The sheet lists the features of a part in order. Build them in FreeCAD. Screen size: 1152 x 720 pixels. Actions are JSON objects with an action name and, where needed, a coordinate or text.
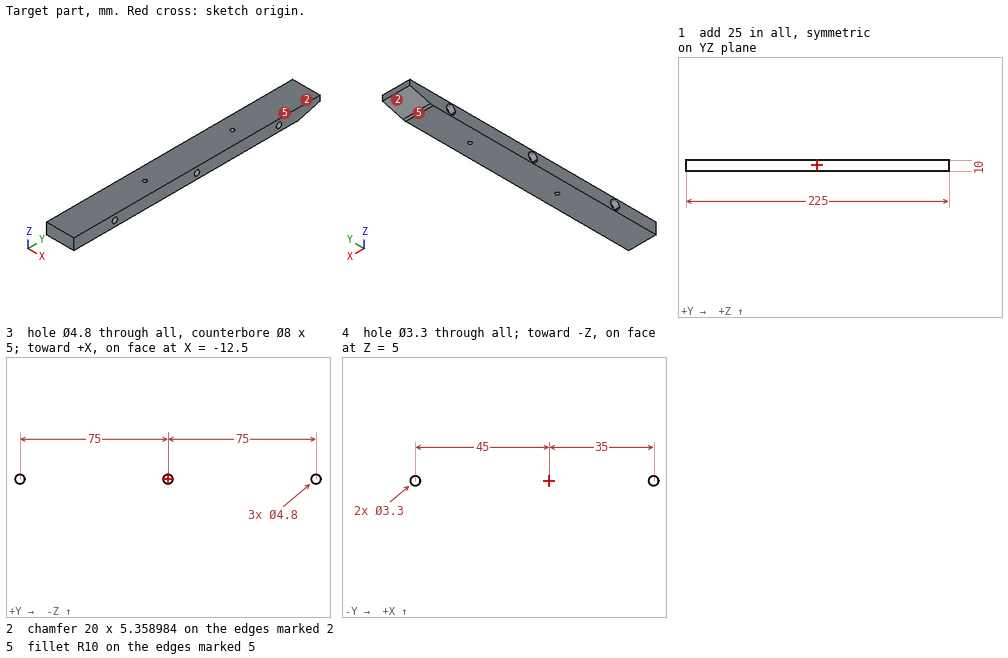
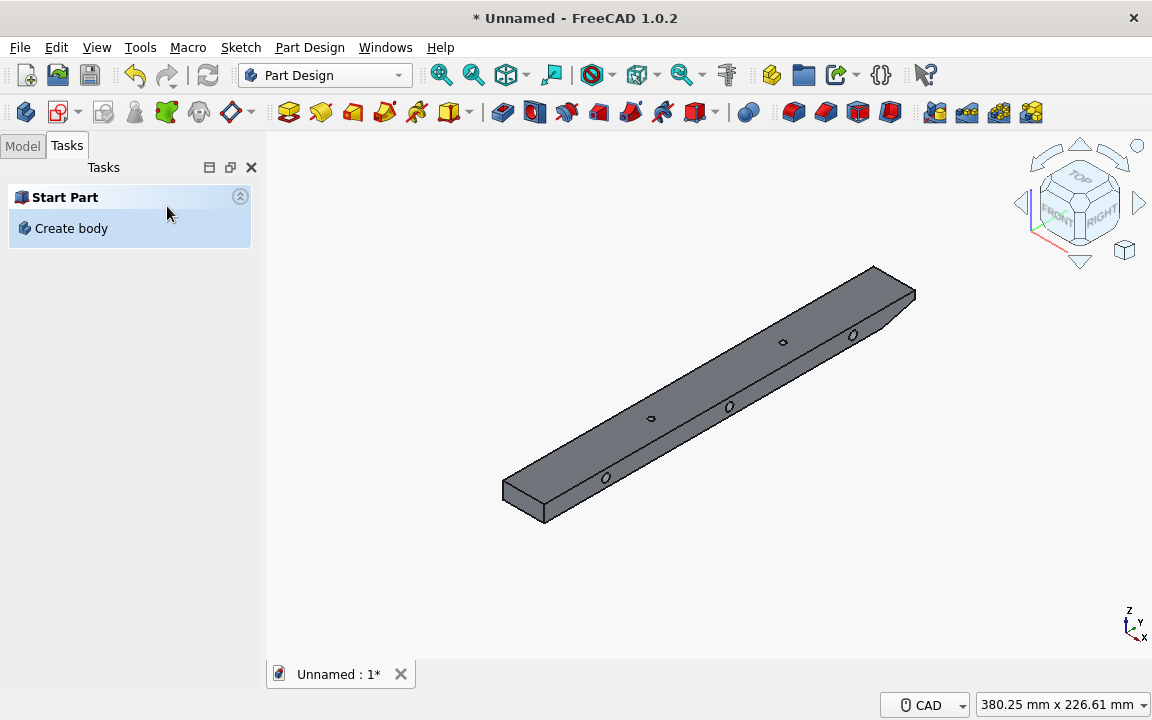
{"action": "key", "text": "2"}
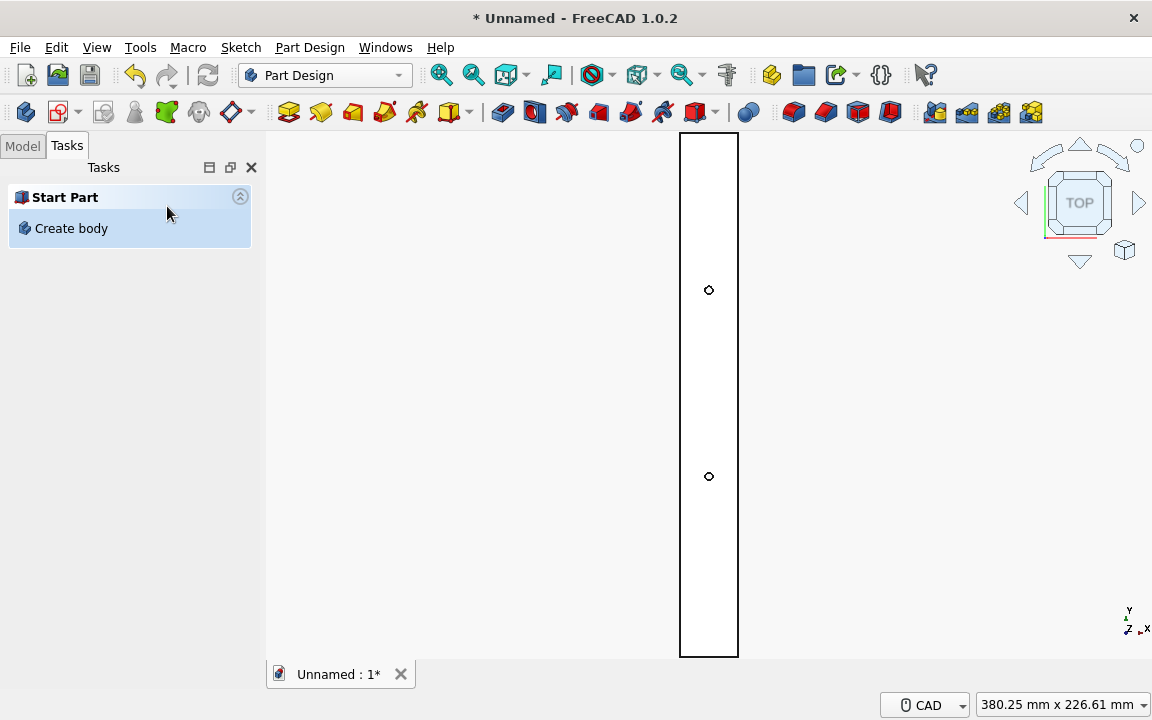
{"action": "key", "text": "0"}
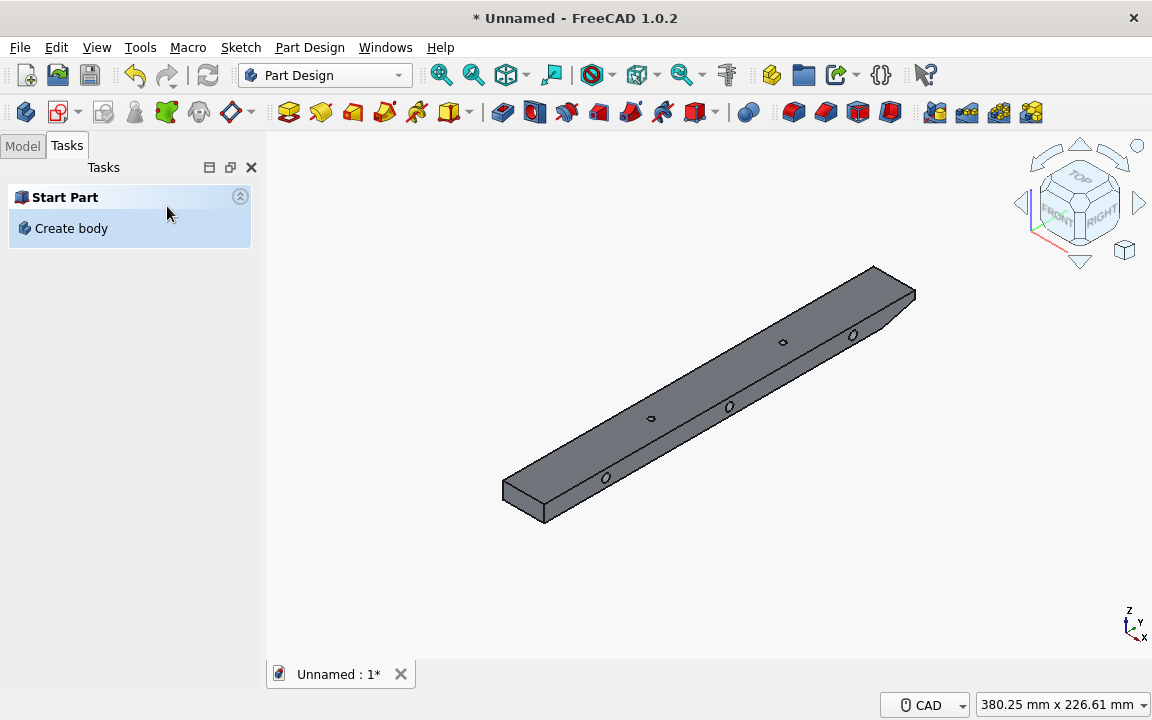
{"action": "key", "text": "1"}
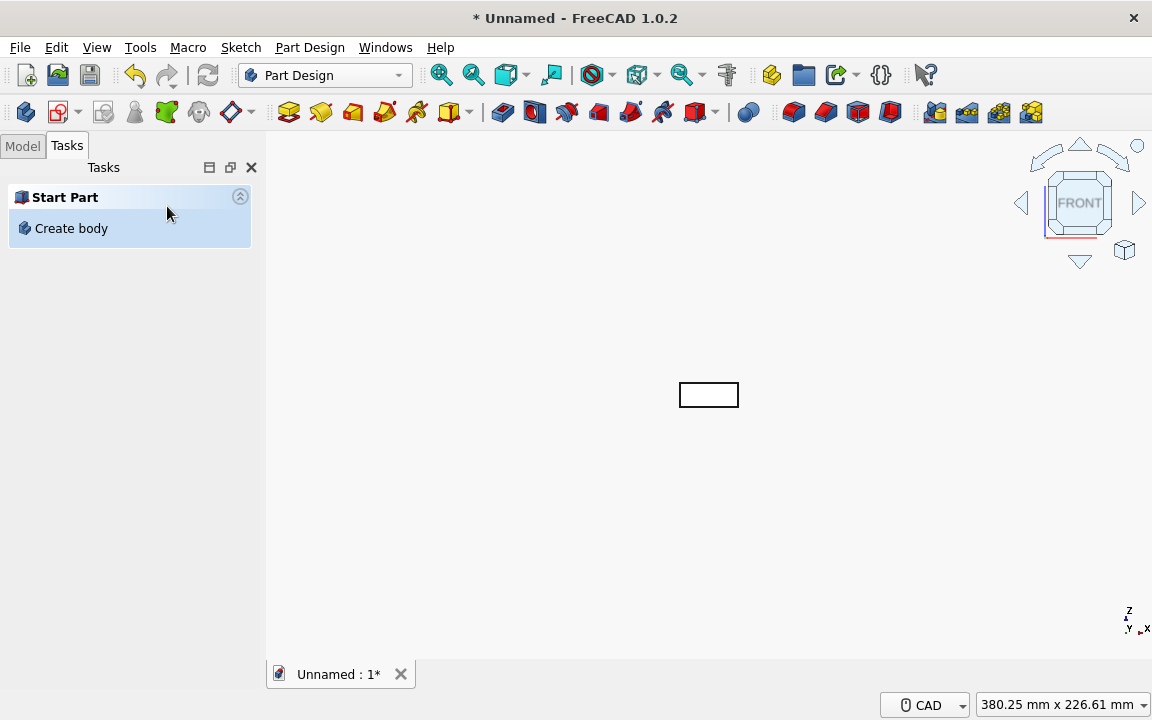
{"action": "left_click", "coordinate": [442, 76]}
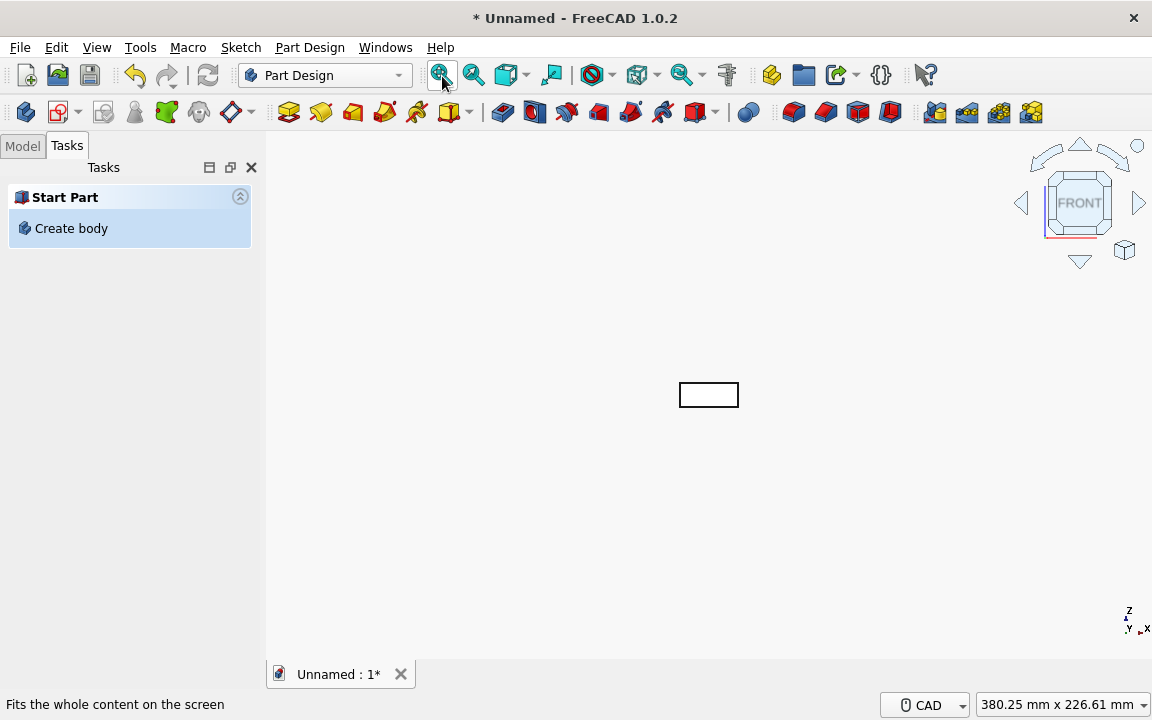
{"action": "key", "text": "3"}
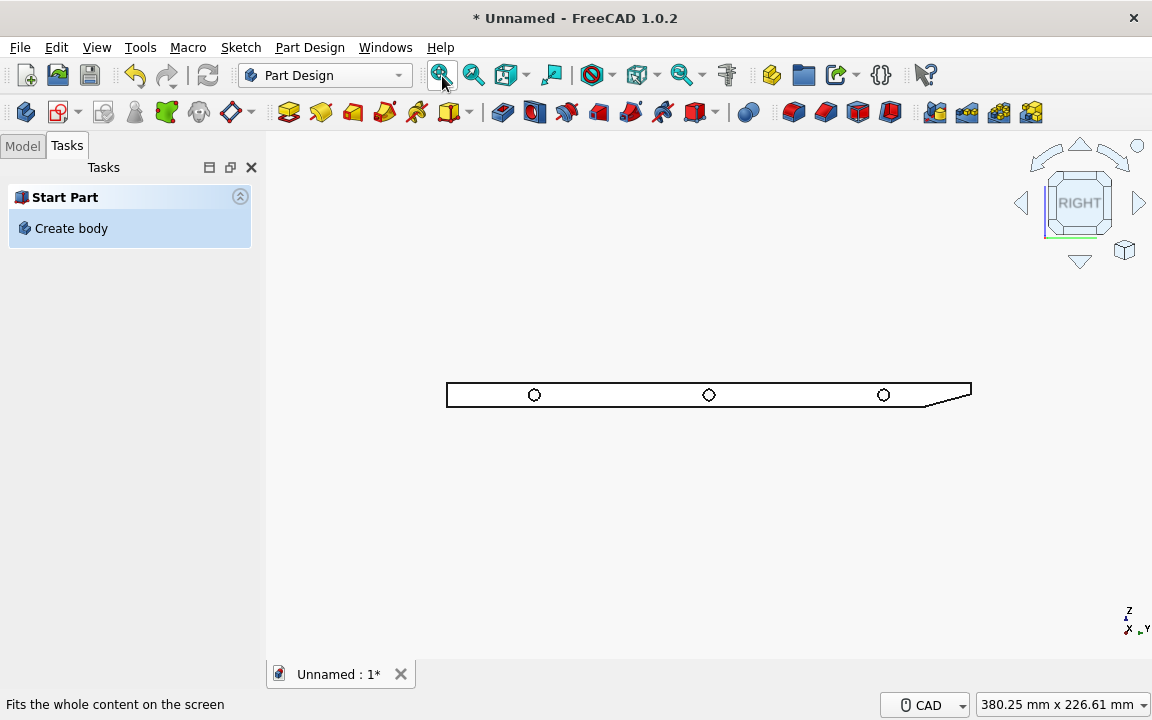
{"action": "key", "text": "5"}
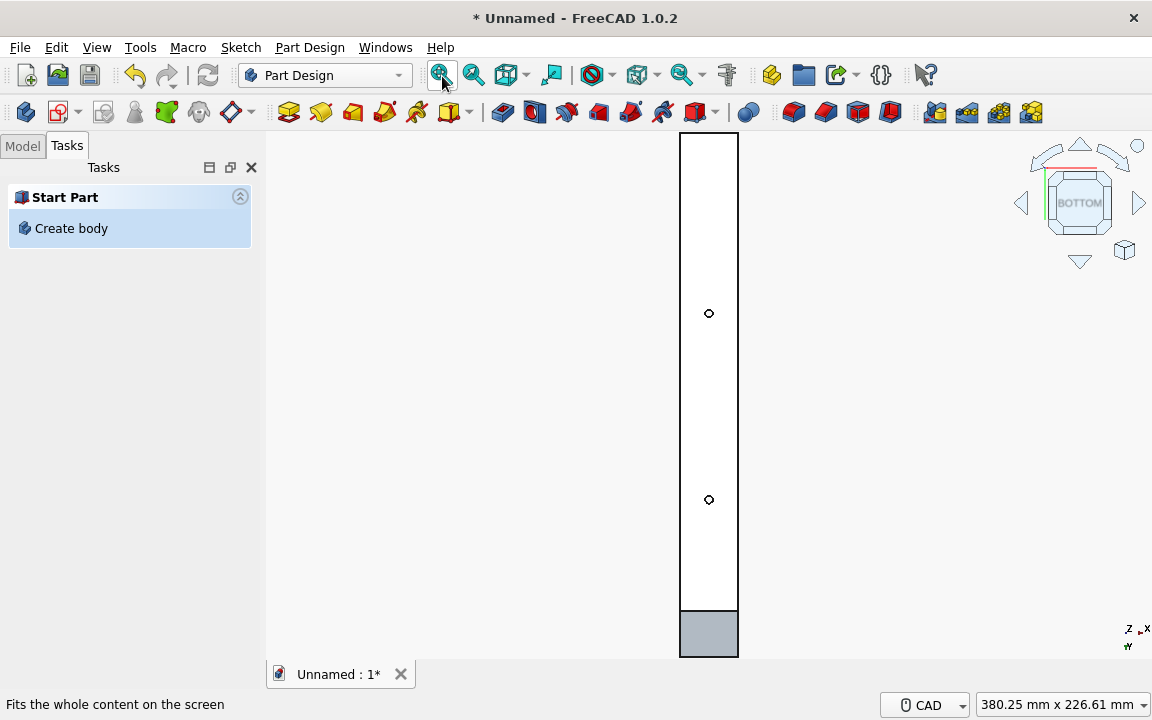
{"action": "left_click", "coordinate": [709, 610]}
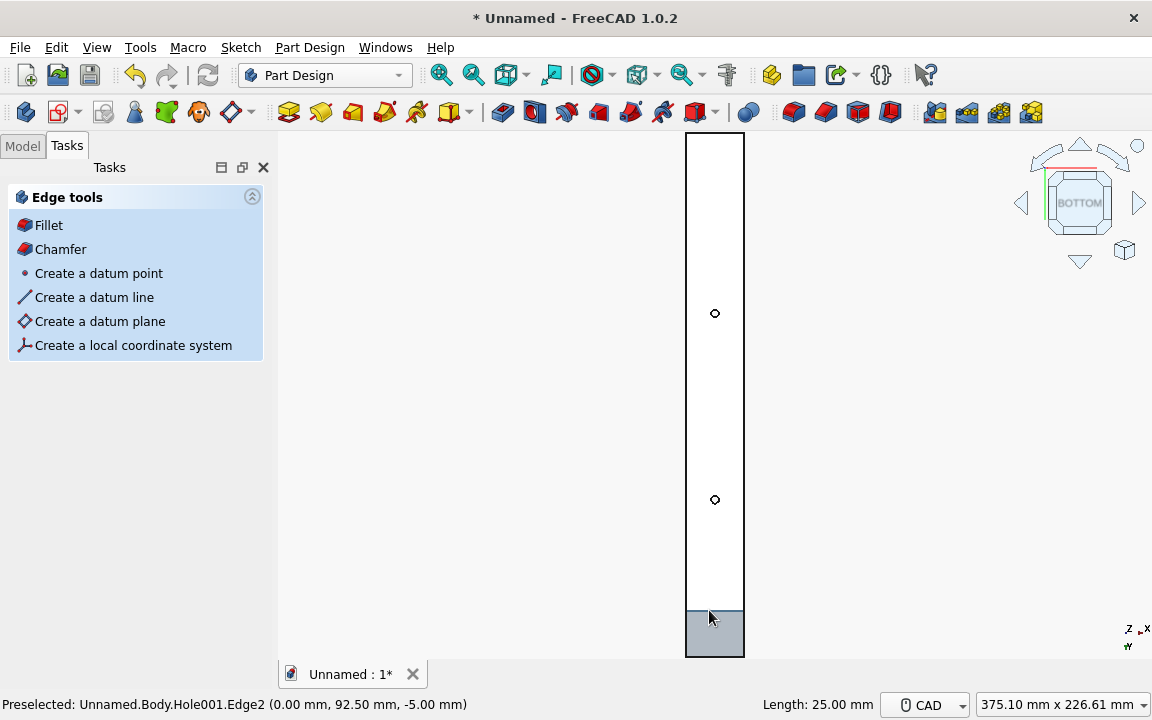
{"action": "left_click", "coordinate": [794, 112]}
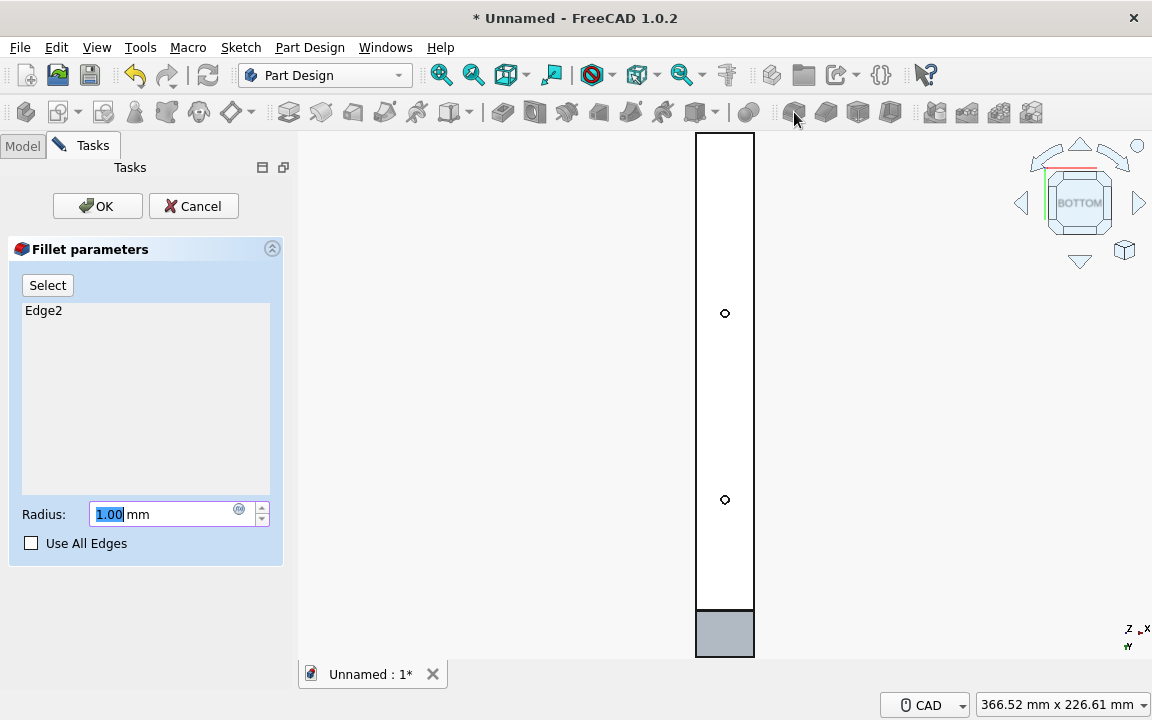
{"action": "type", "text": "10"}
{"action": "key", "text": "Tab"}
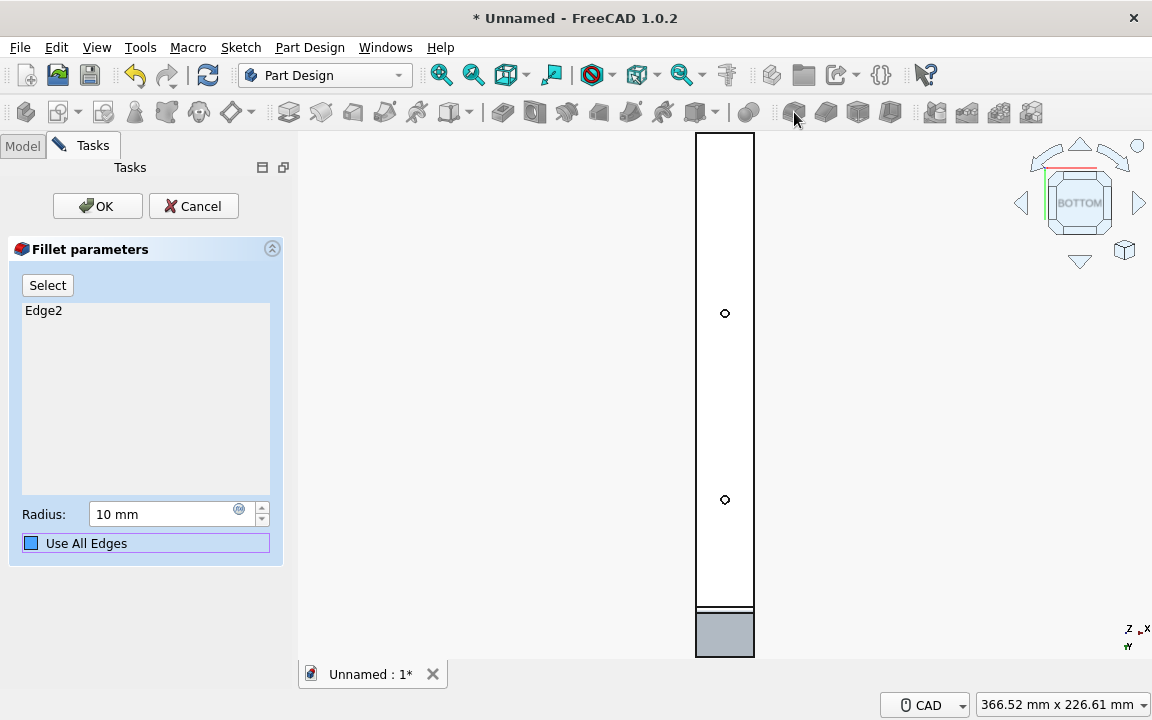
{"action": "left_click", "coordinate": [98, 206]}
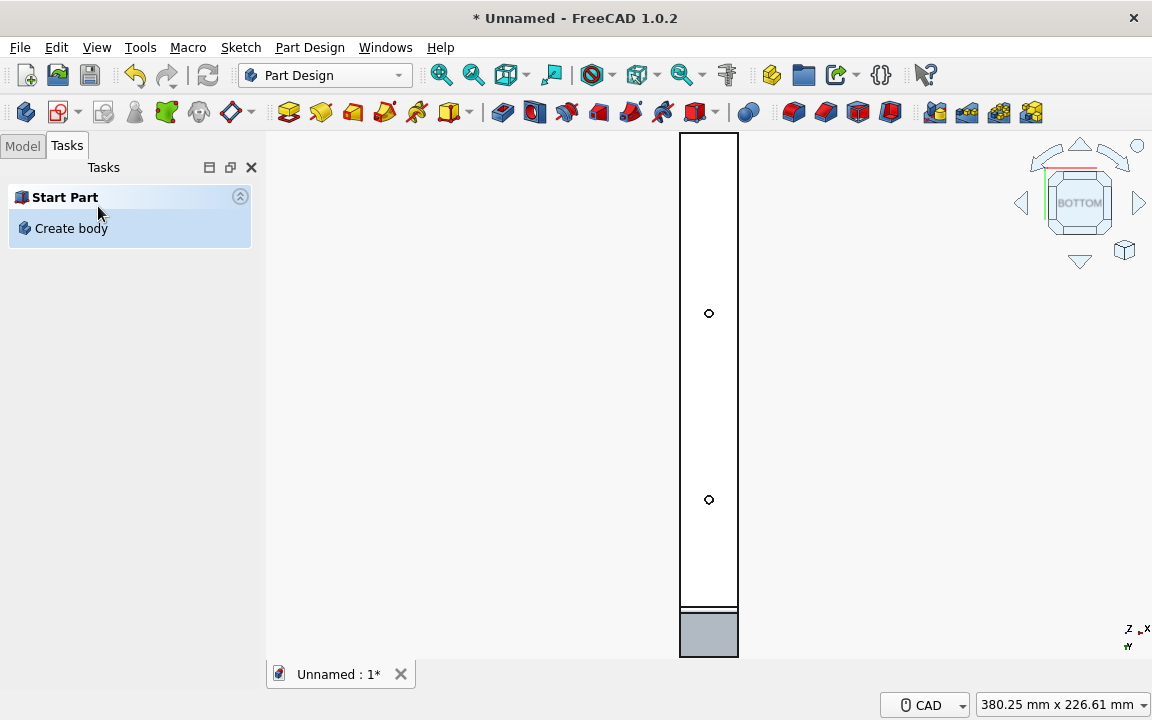
{"action": "key", "text": "0"}